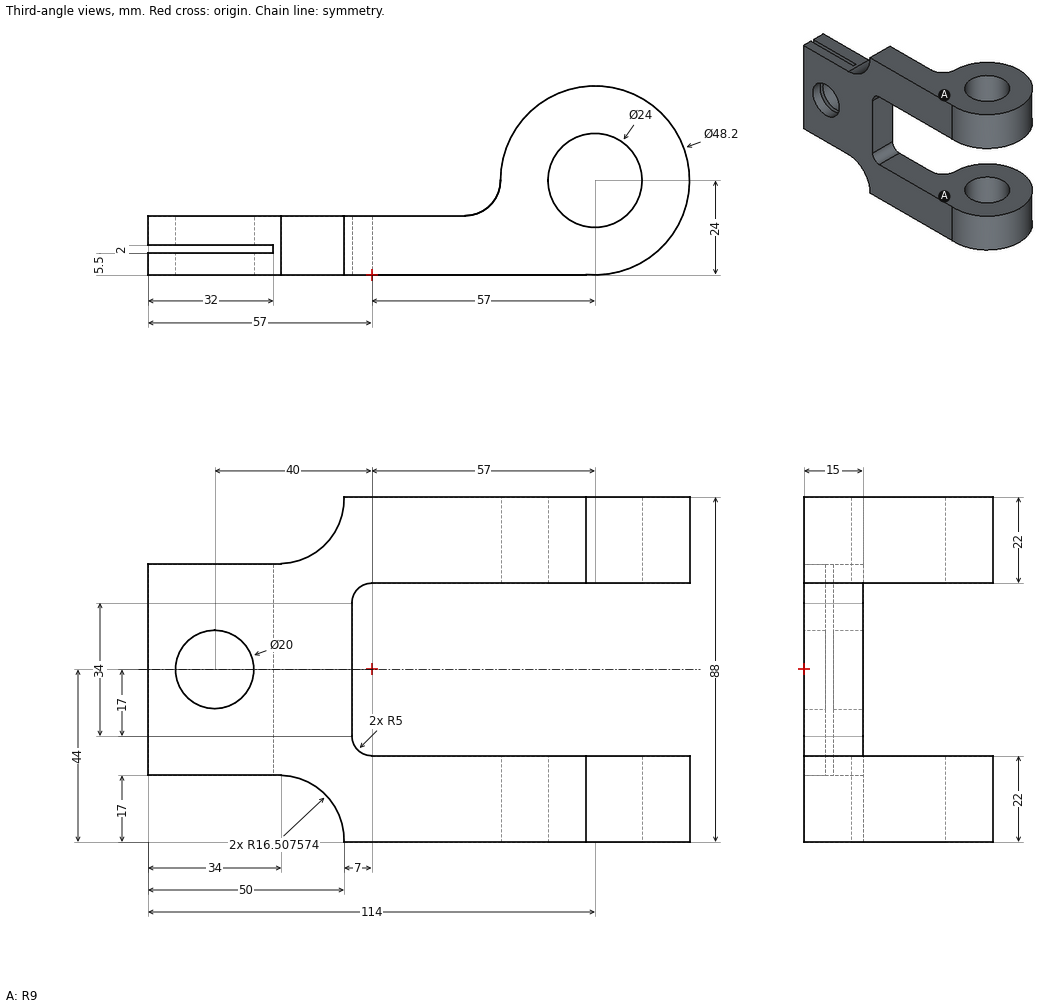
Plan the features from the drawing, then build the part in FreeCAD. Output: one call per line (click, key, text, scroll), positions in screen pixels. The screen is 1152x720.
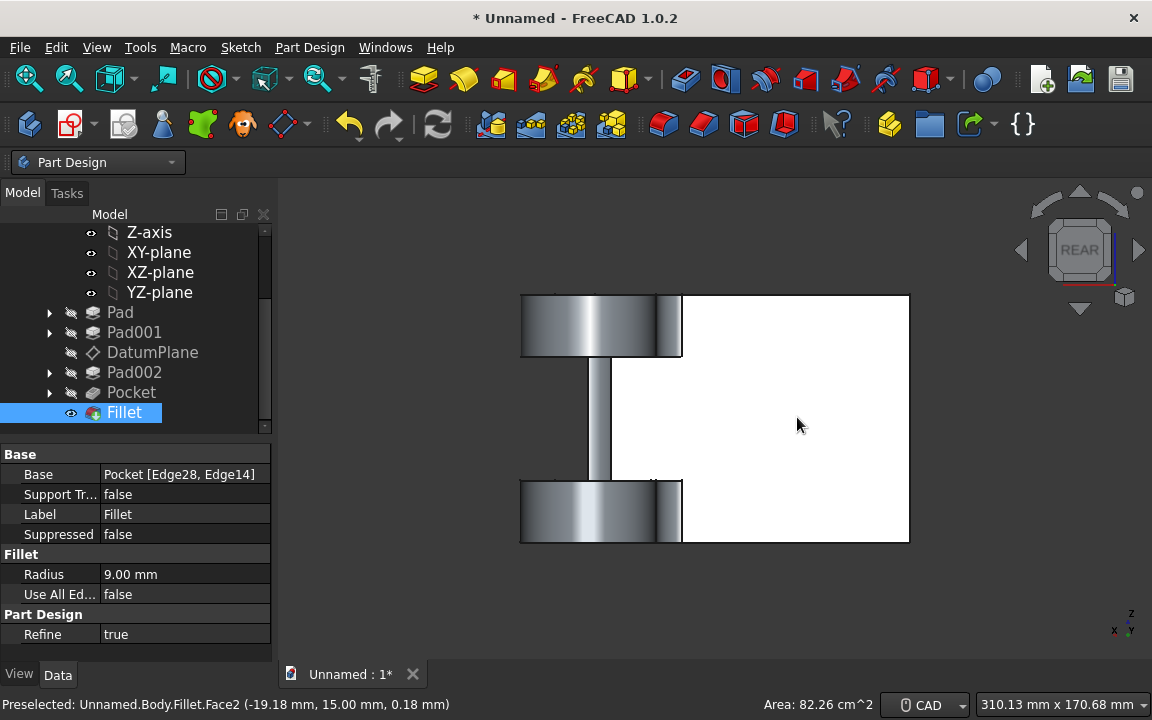
click(70, 124)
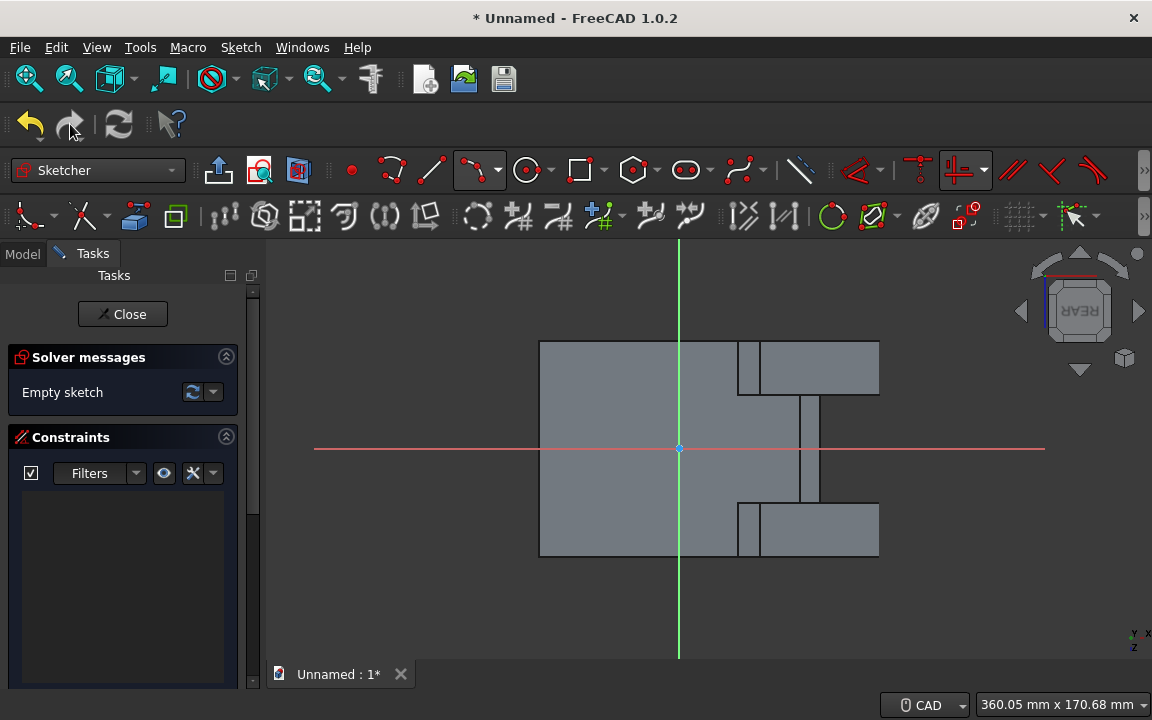
key(q)
key(s)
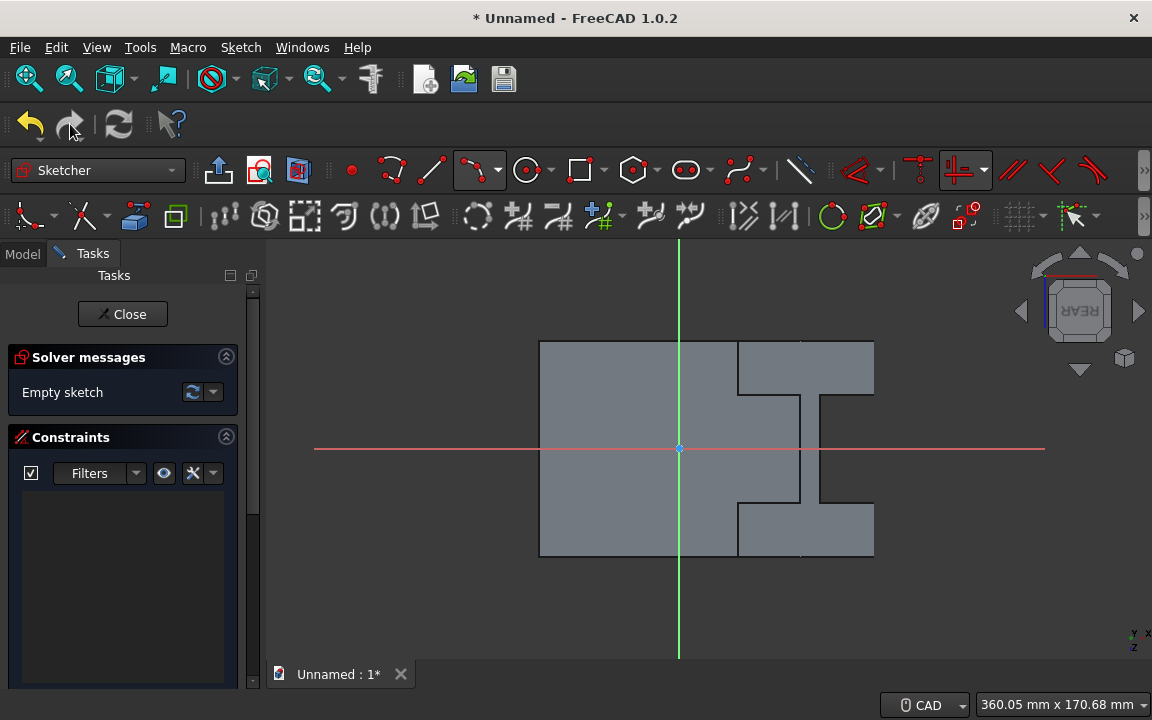
key(g)
key(l)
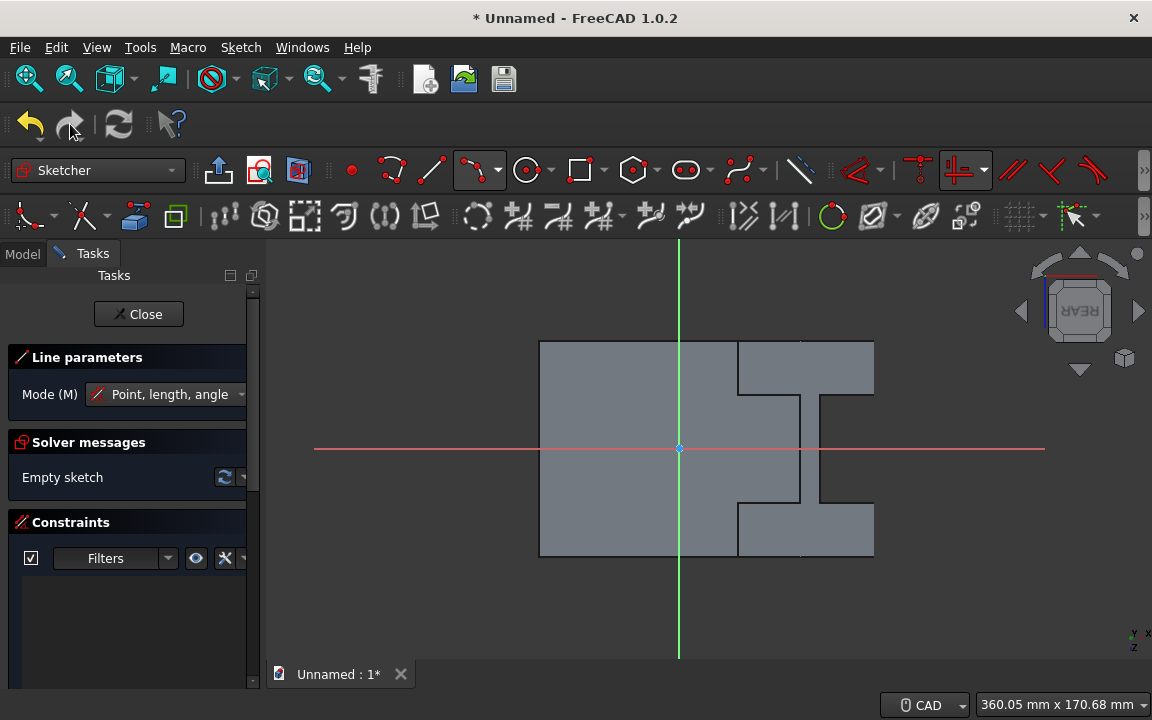
scroll(667, 407, up, 2)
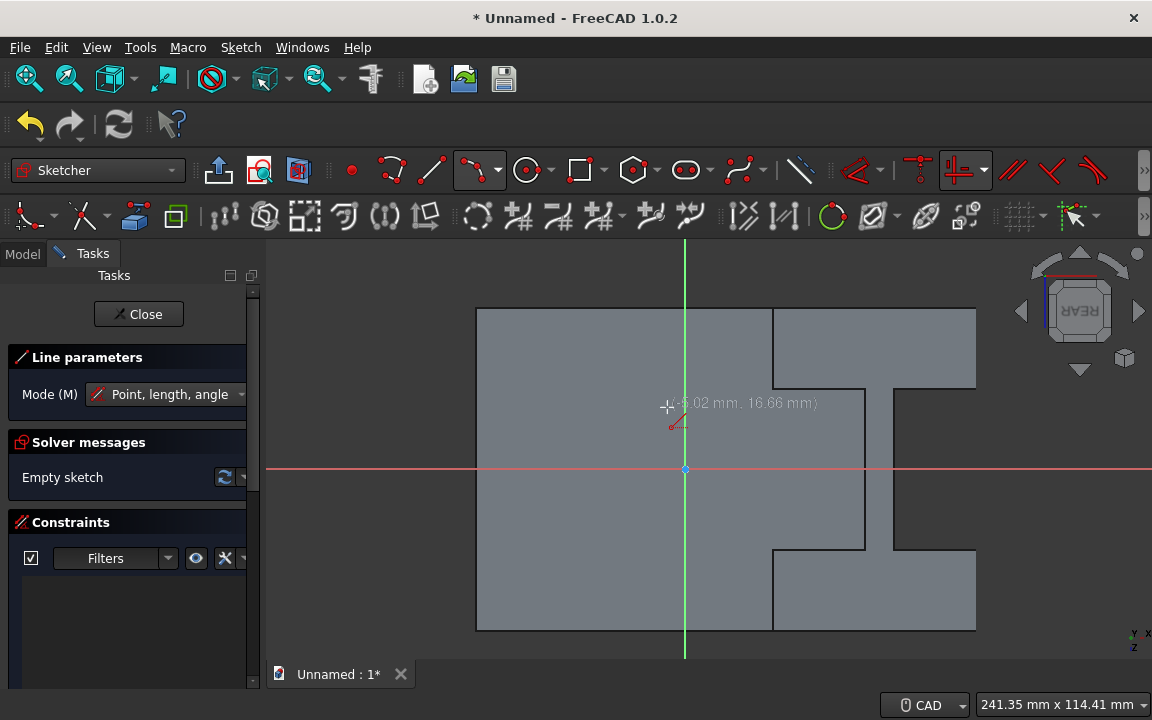
click(667, 407)
click(667, 532)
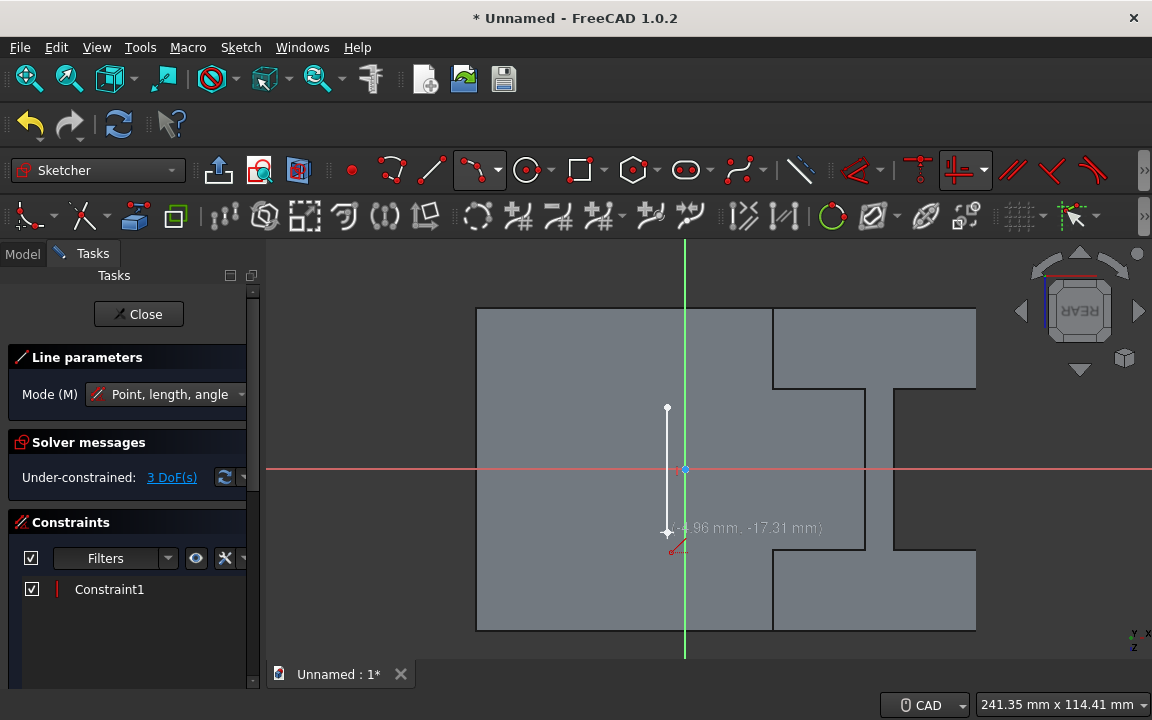
click(392, 170)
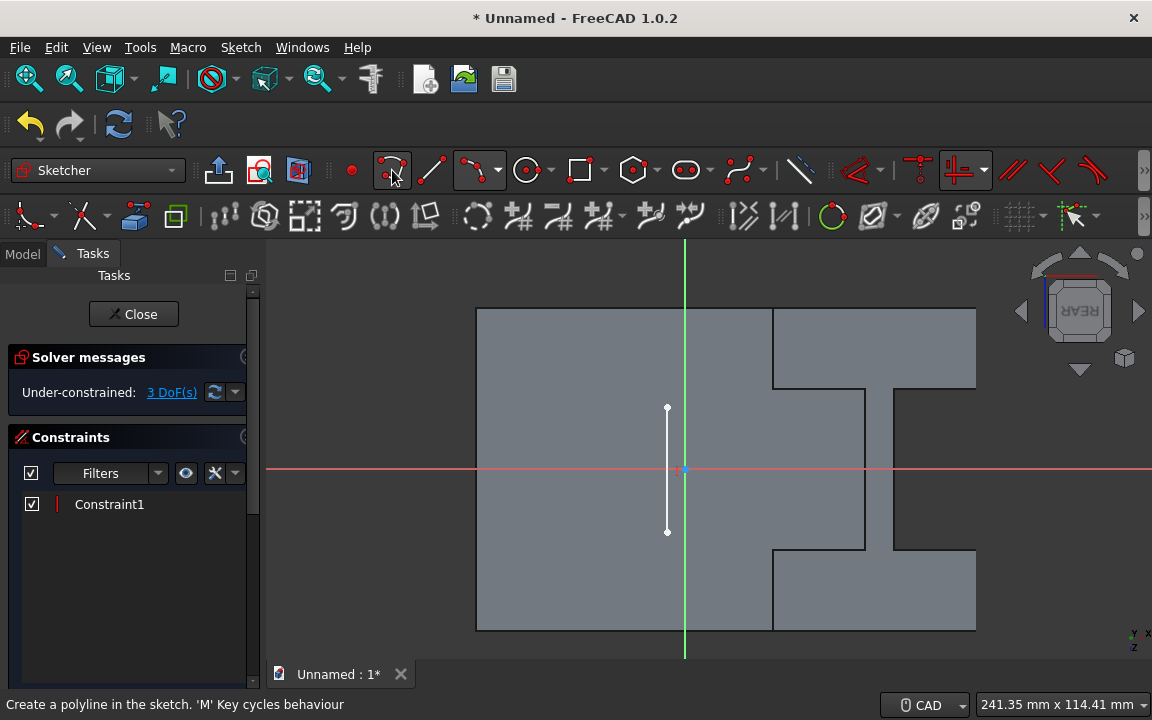
click(685, 550)
click(894, 550)
click(894, 389)
click(685, 389)
right_click(685, 389)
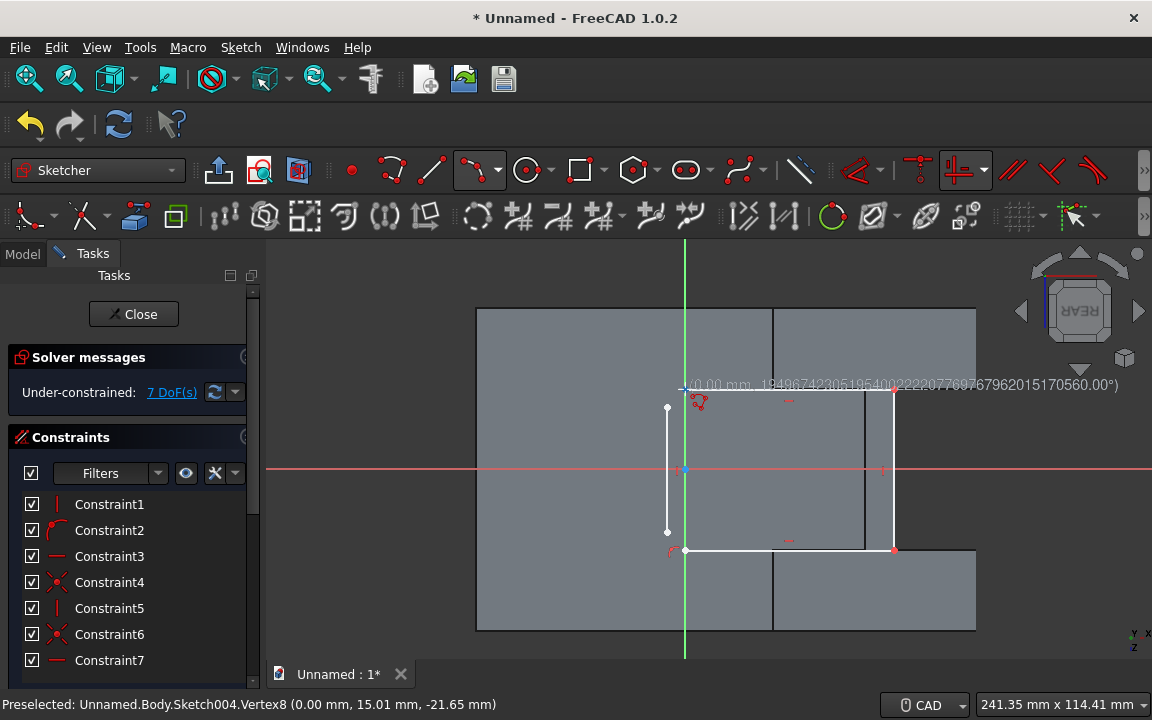
key(g)
key(3)
key(a)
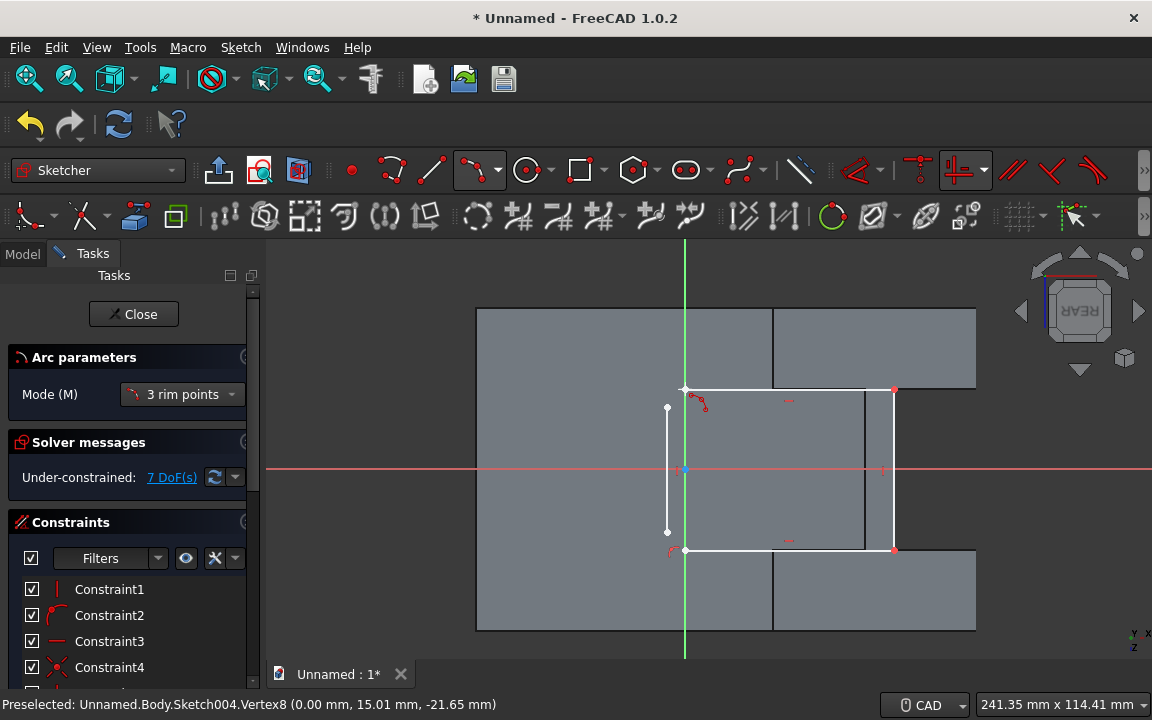
click(667, 533)
click(685, 551)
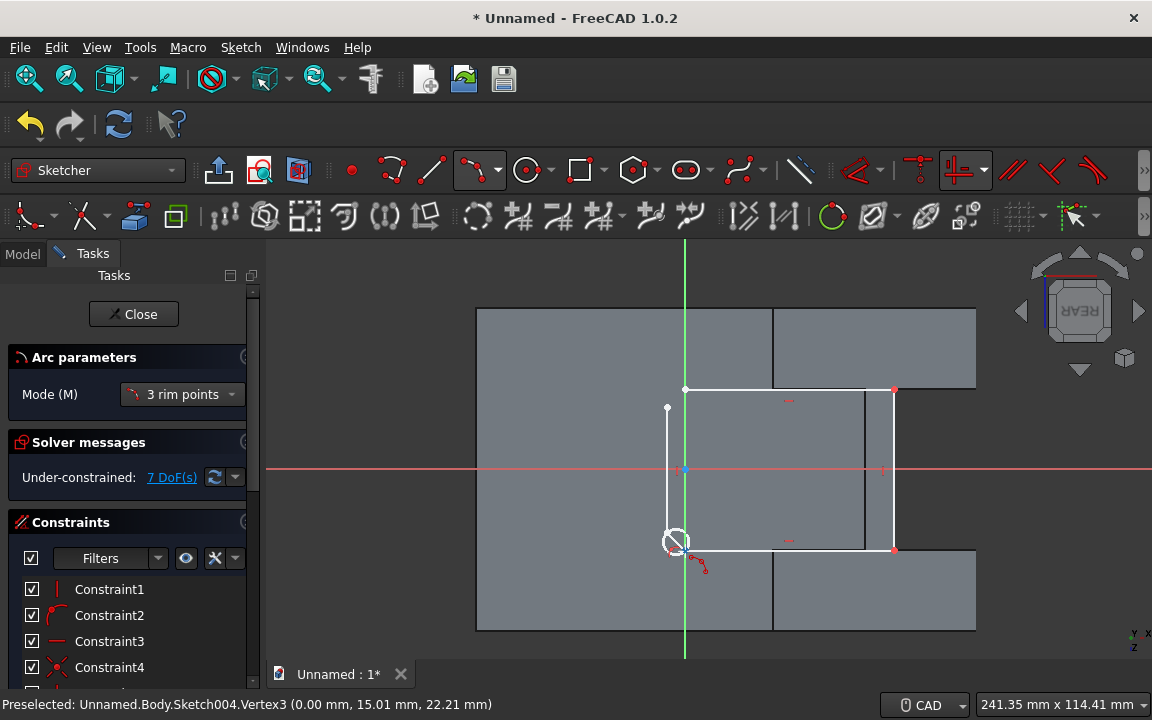
scroll(672, 545, up, 6)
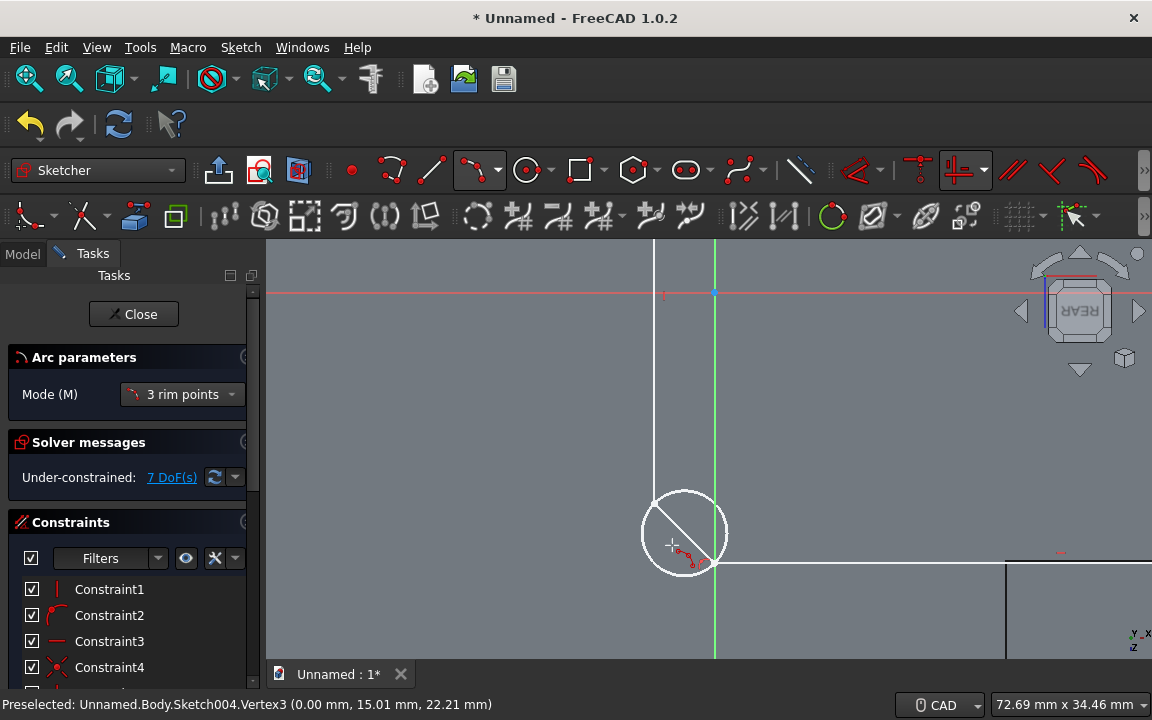
click(672, 543)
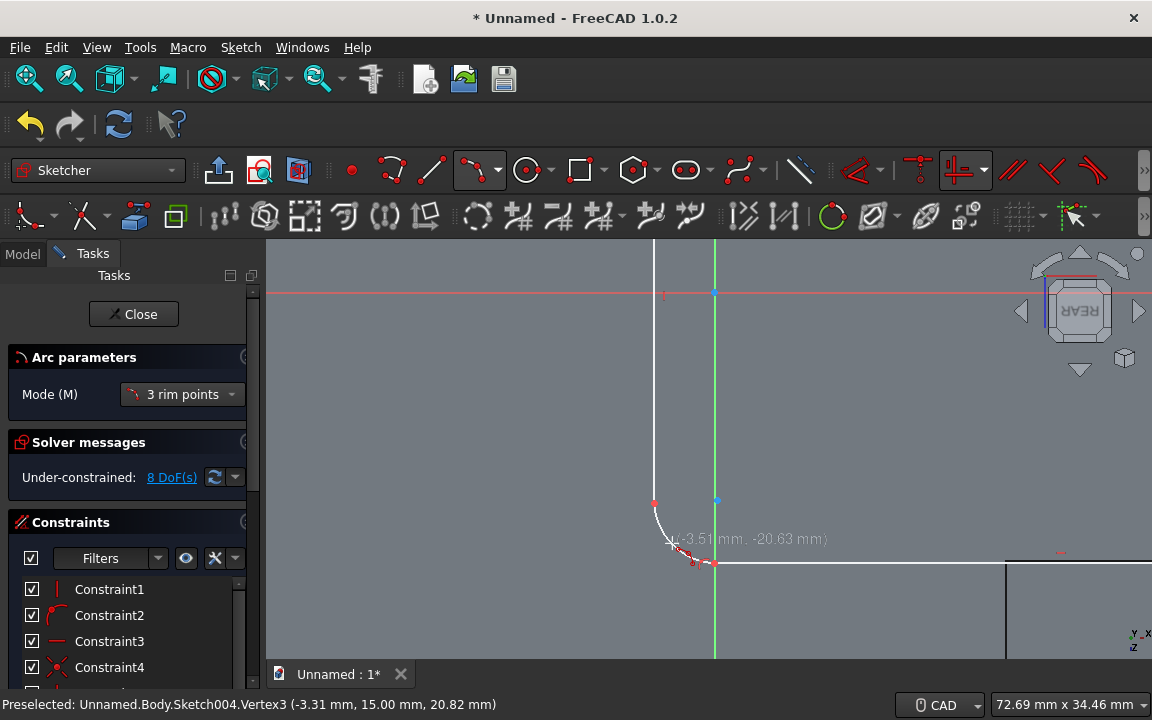
scroll(616, 500, down, 7)